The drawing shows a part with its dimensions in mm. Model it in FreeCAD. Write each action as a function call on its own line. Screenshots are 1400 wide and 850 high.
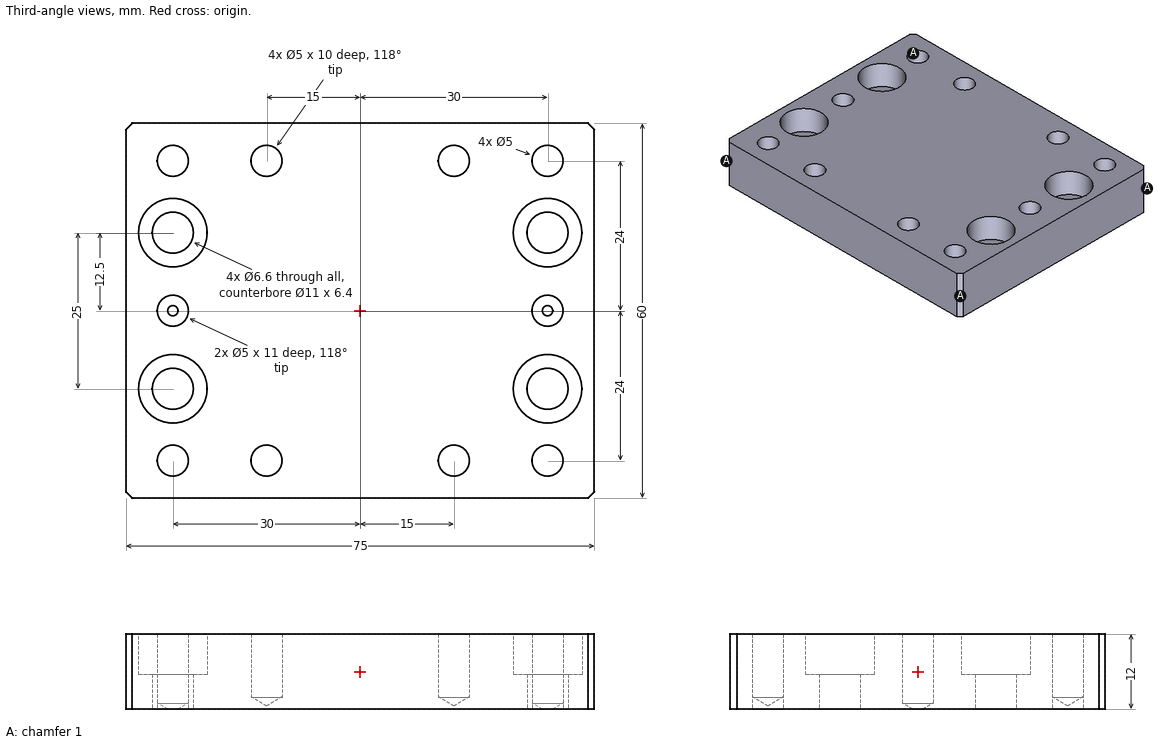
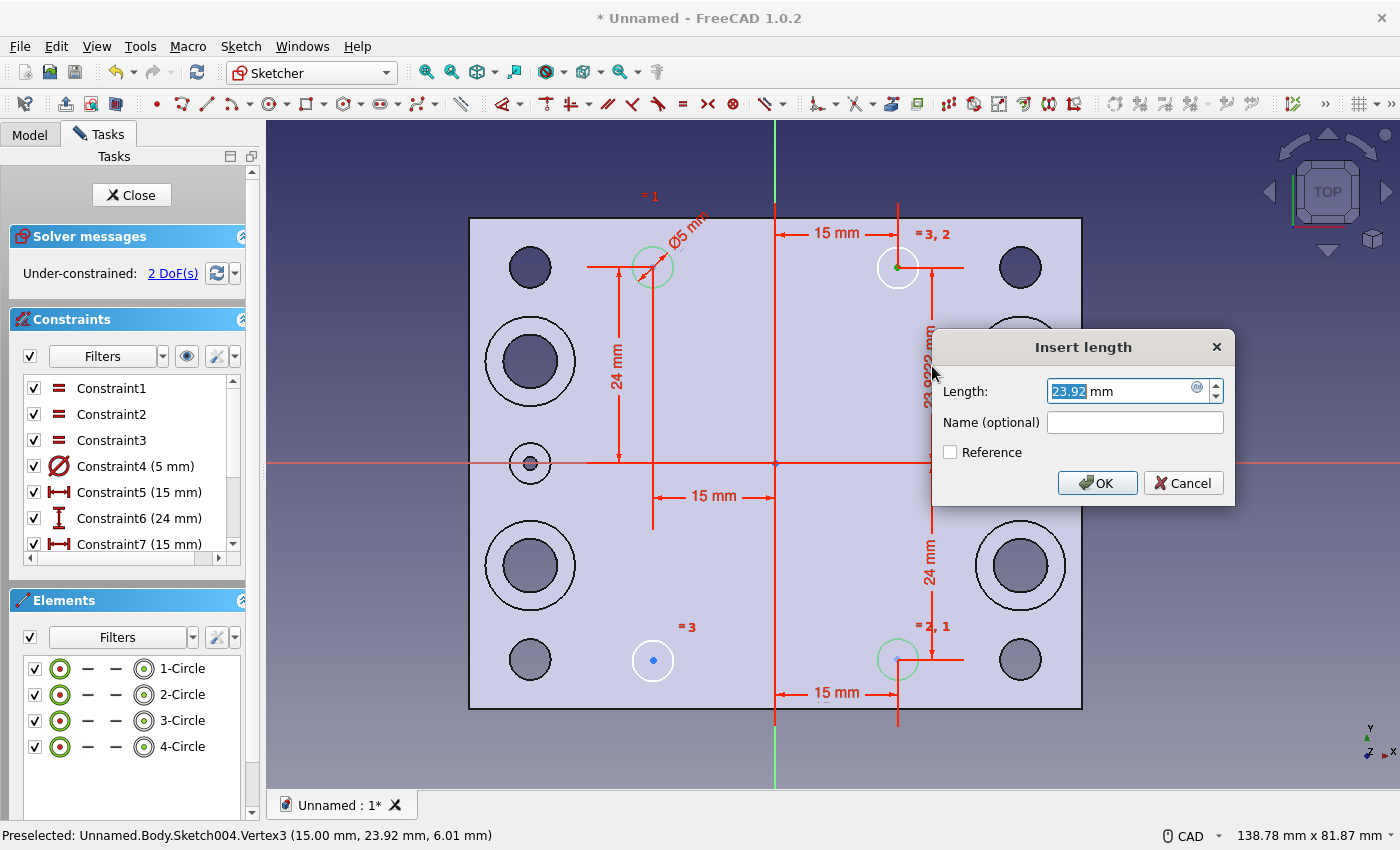
text(24)
key(Return)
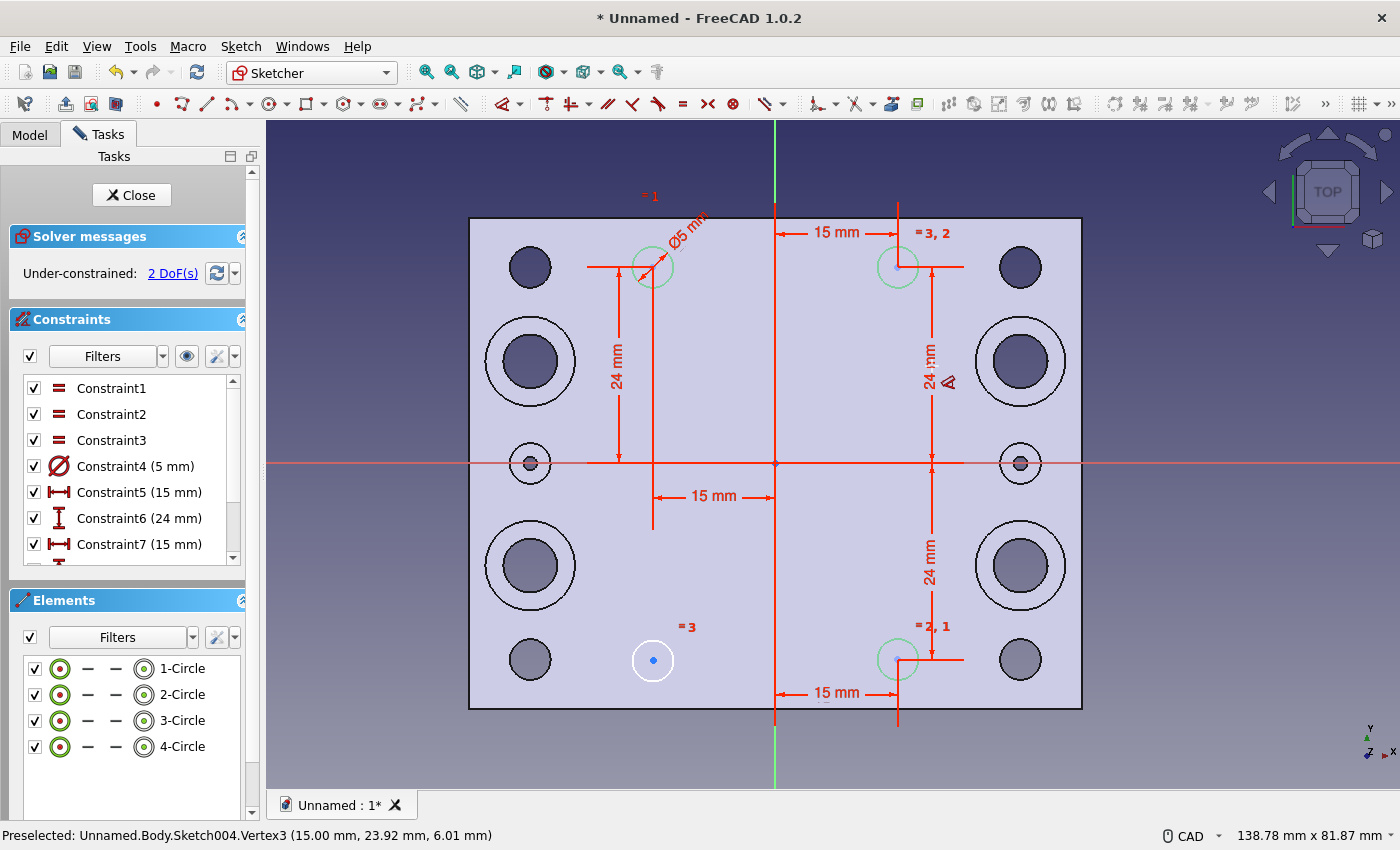
click(653, 661)
click(714, 695)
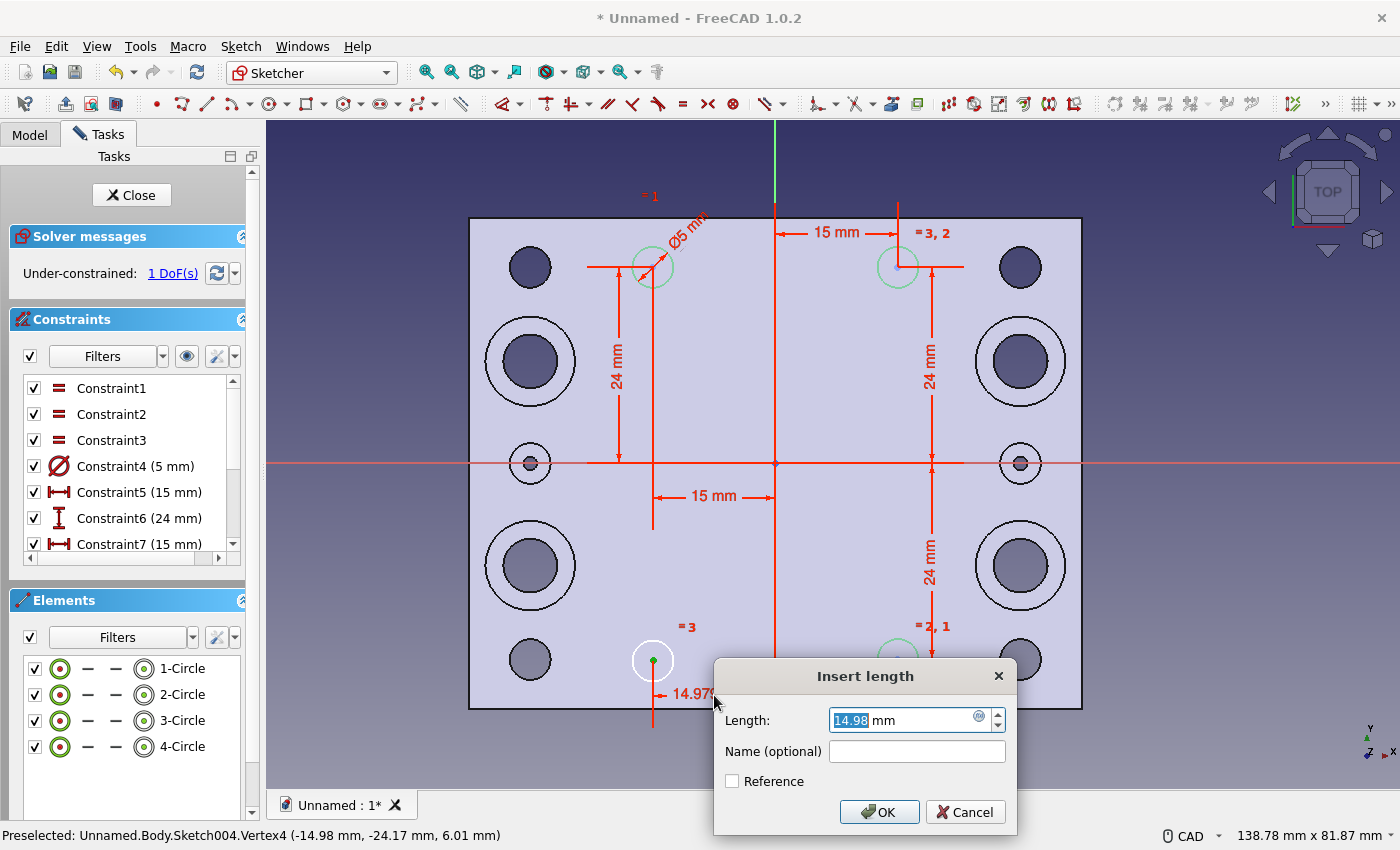
text(15)
key(Return)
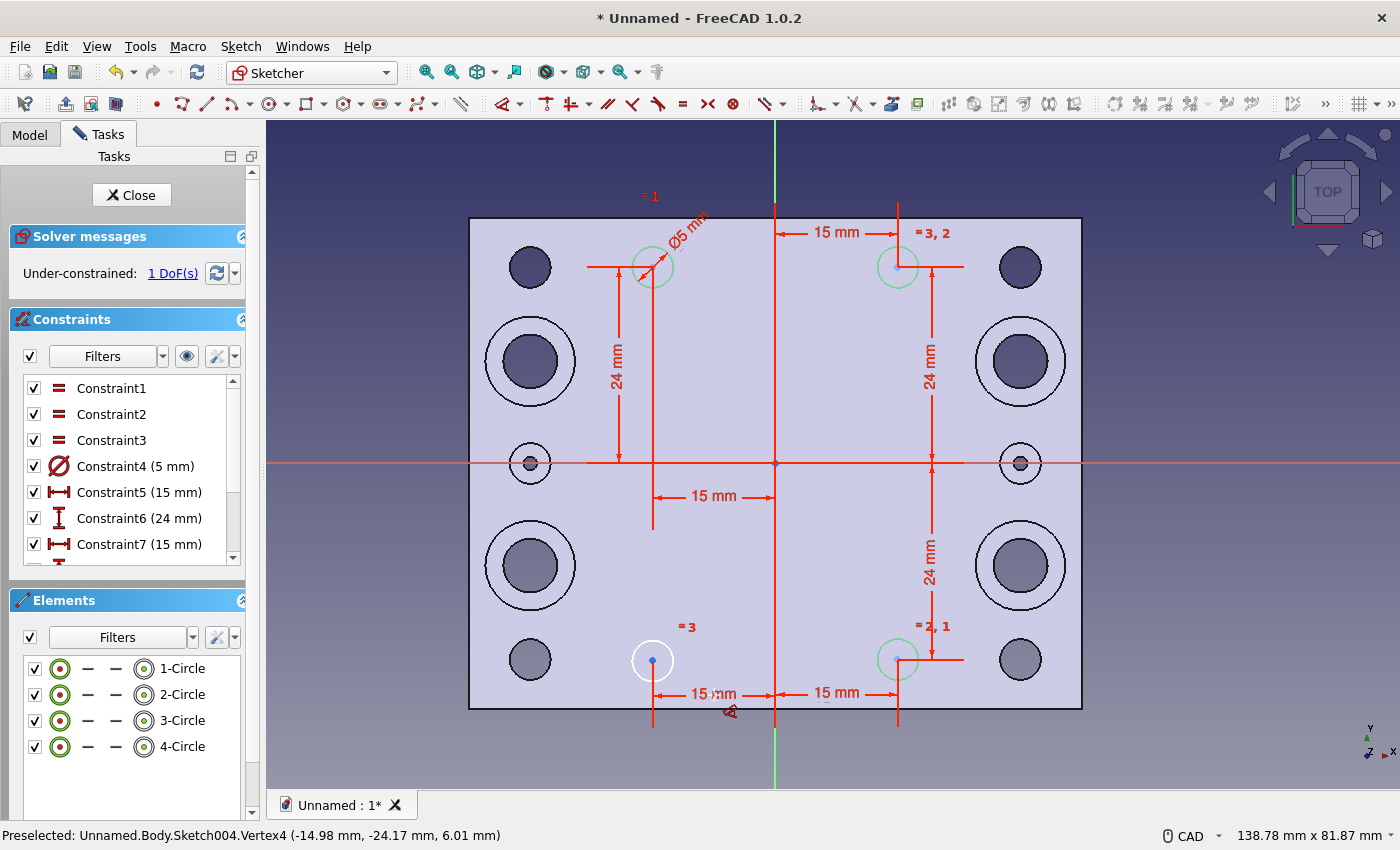
click(653, 661)
click(619, 562)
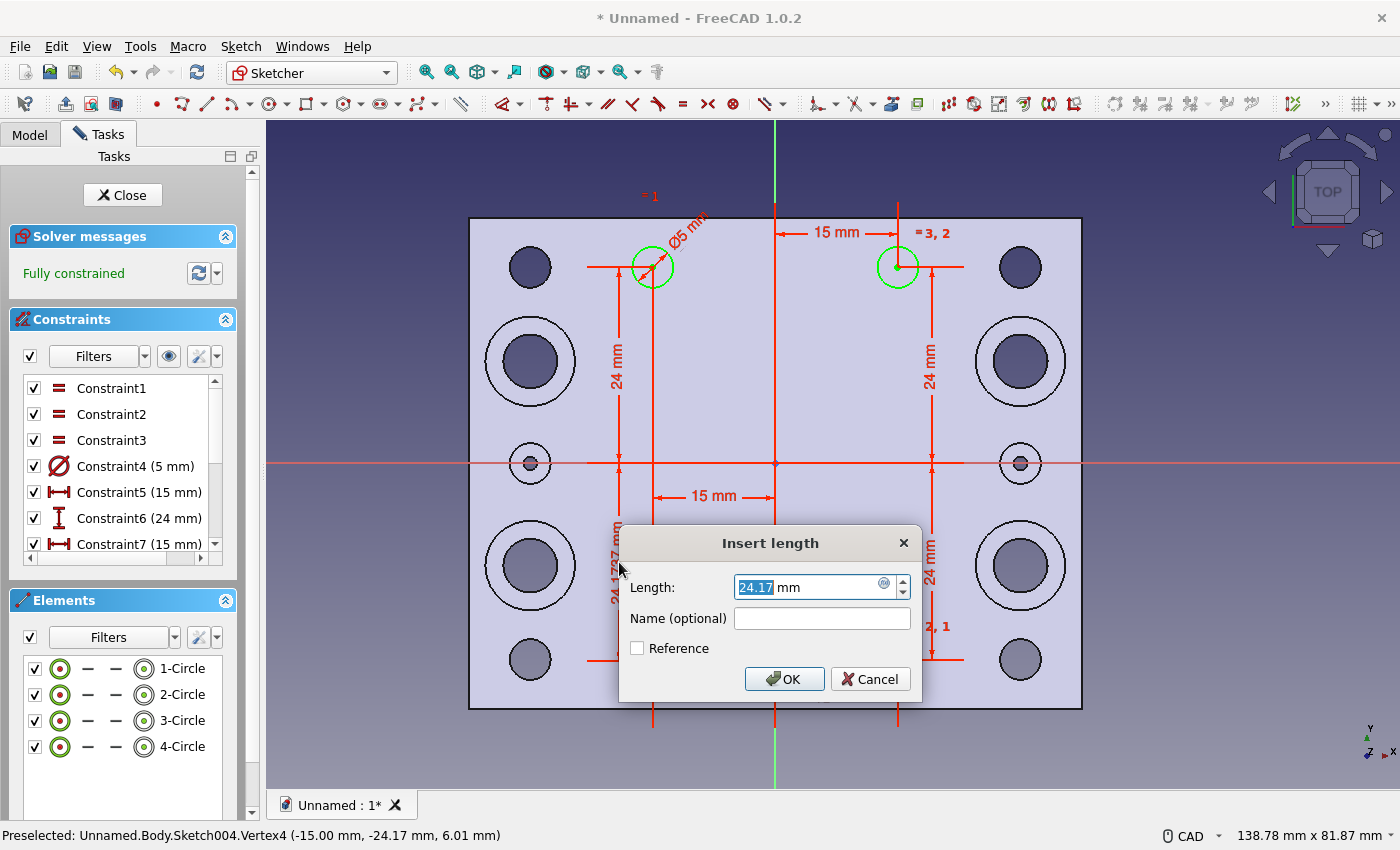
text(24)
key(Return)
key(Escape)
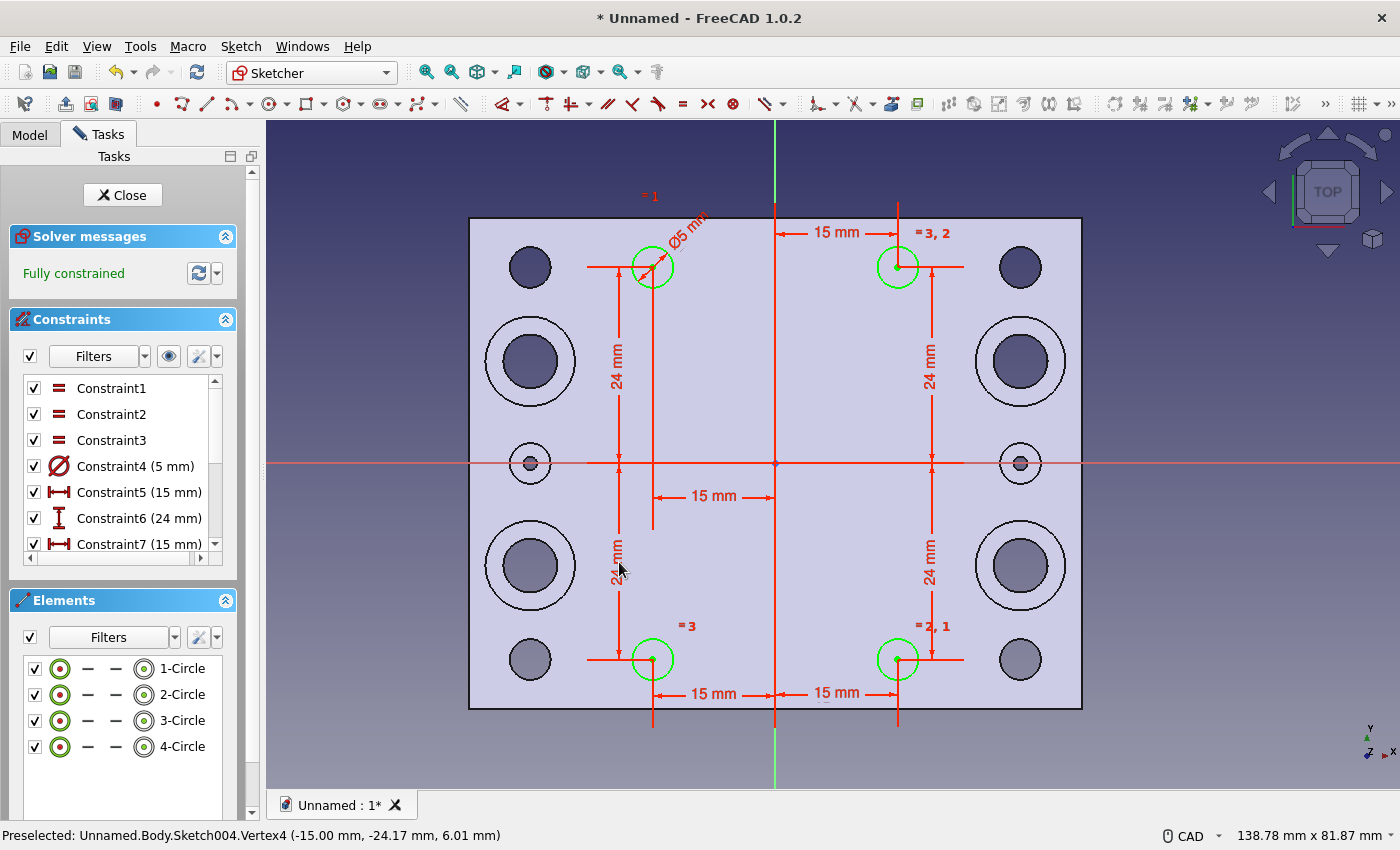
click(123, 195)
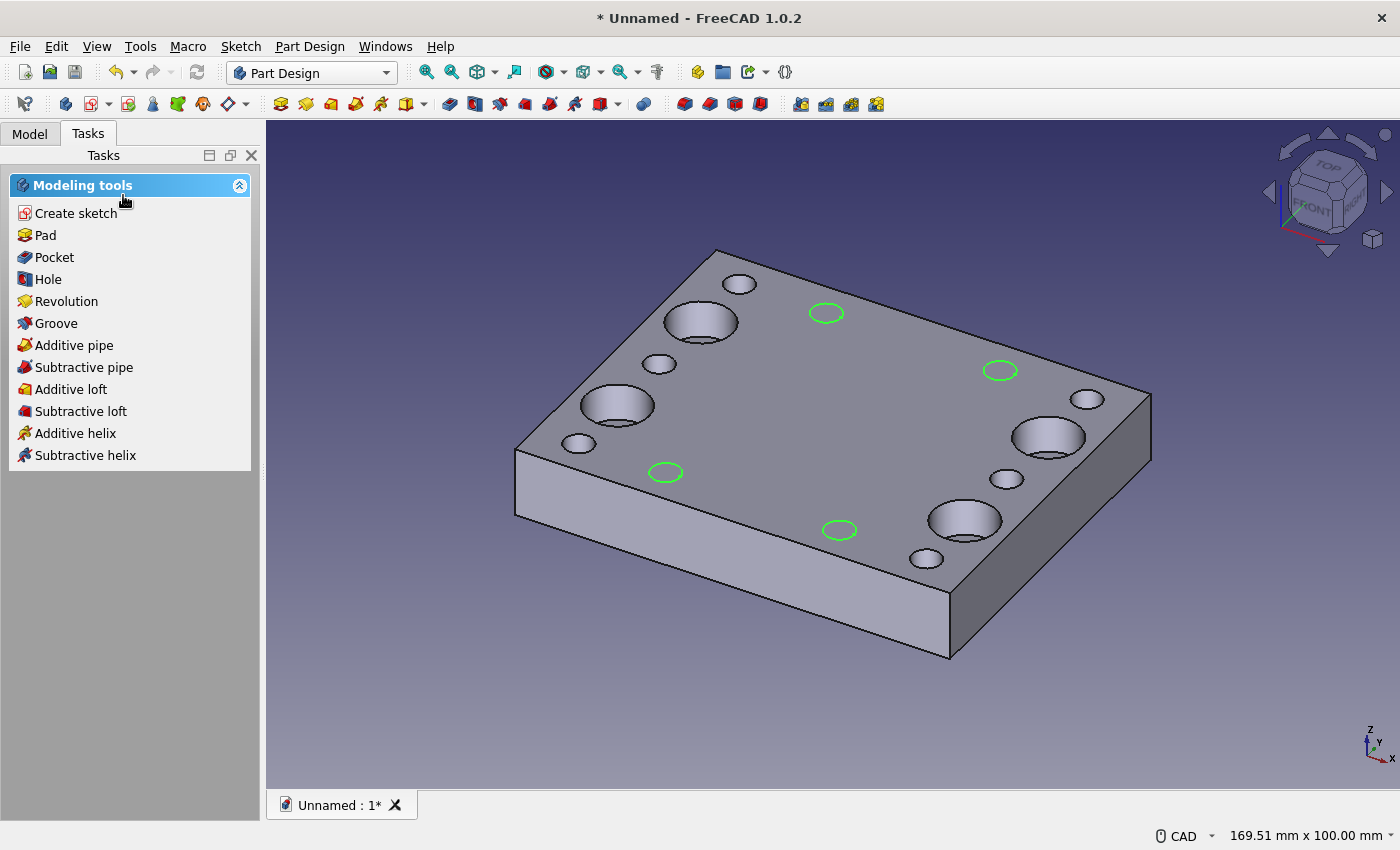
click(475, 104)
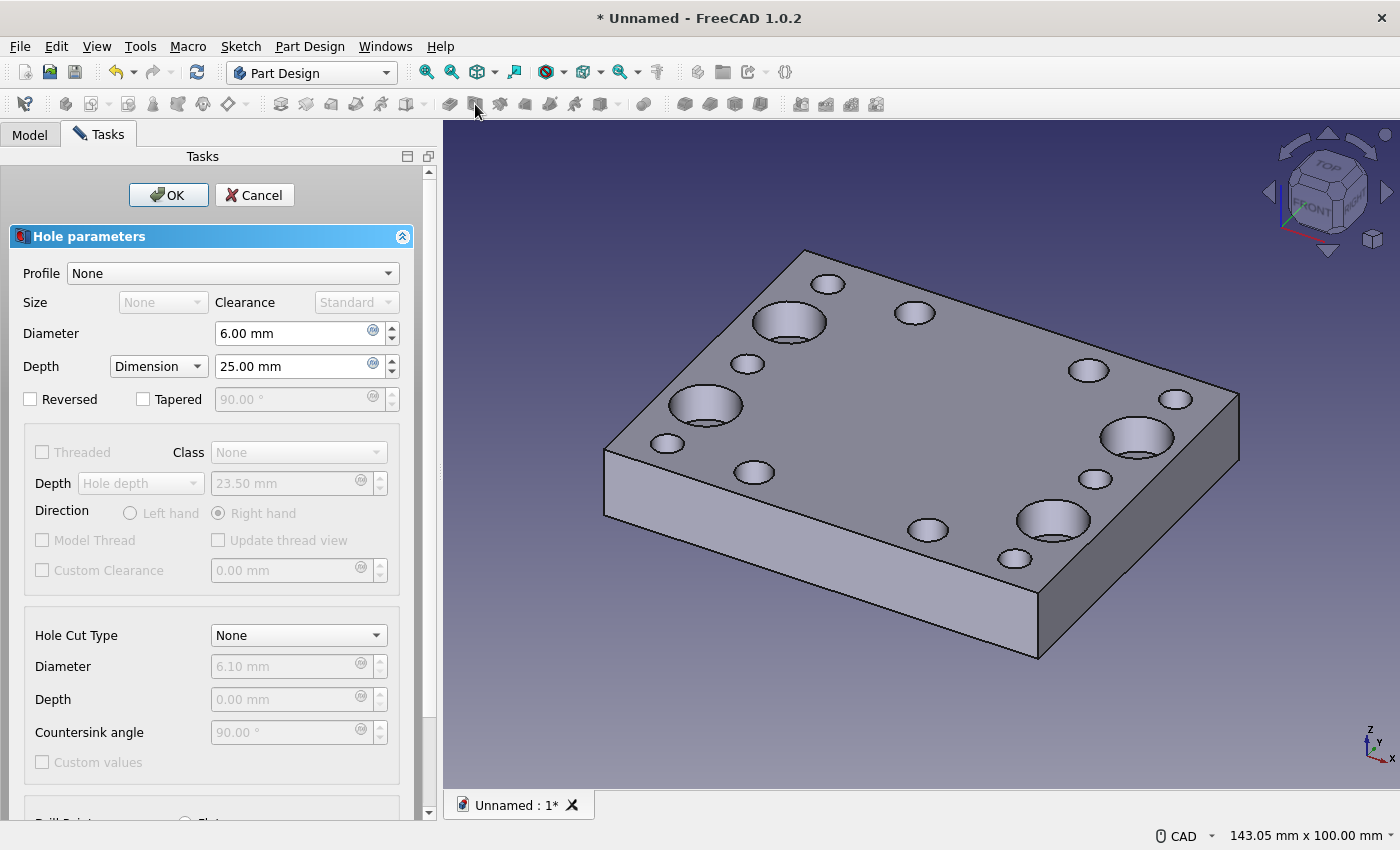
triple_click(300, 334)